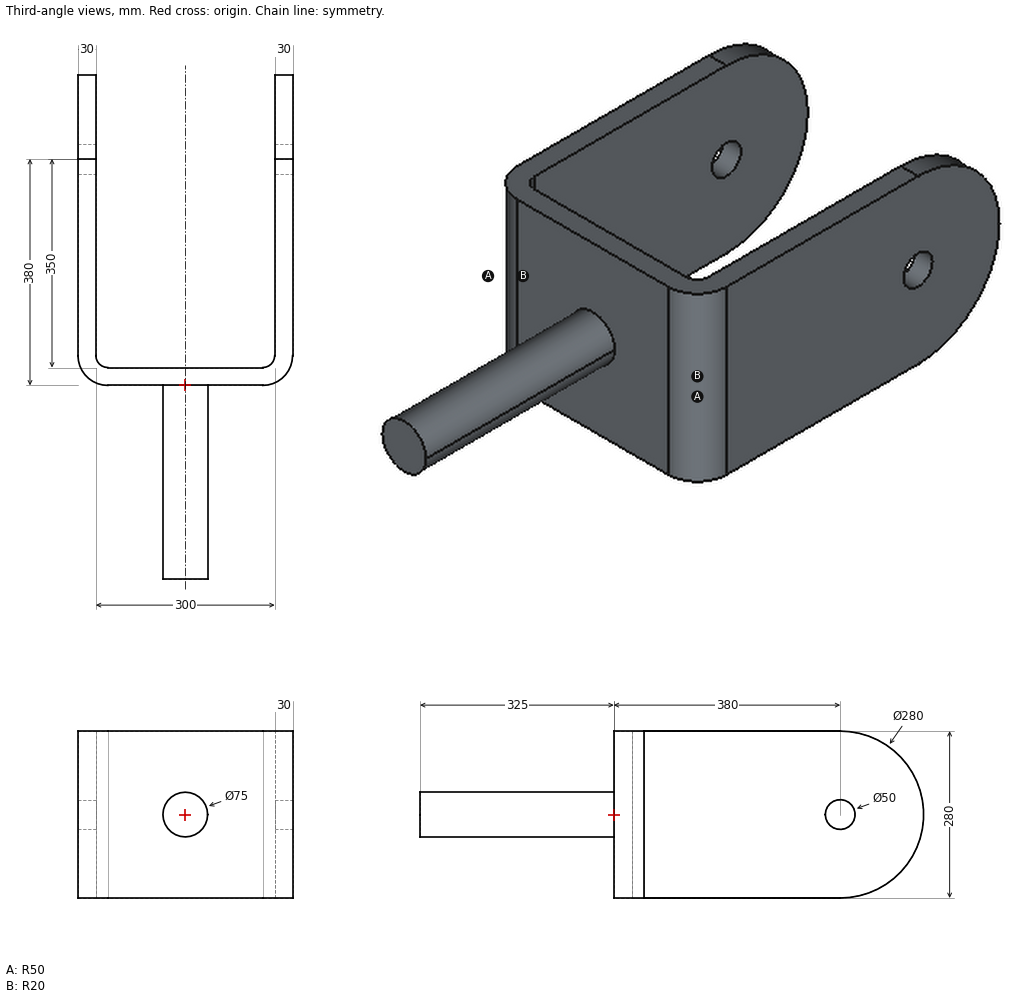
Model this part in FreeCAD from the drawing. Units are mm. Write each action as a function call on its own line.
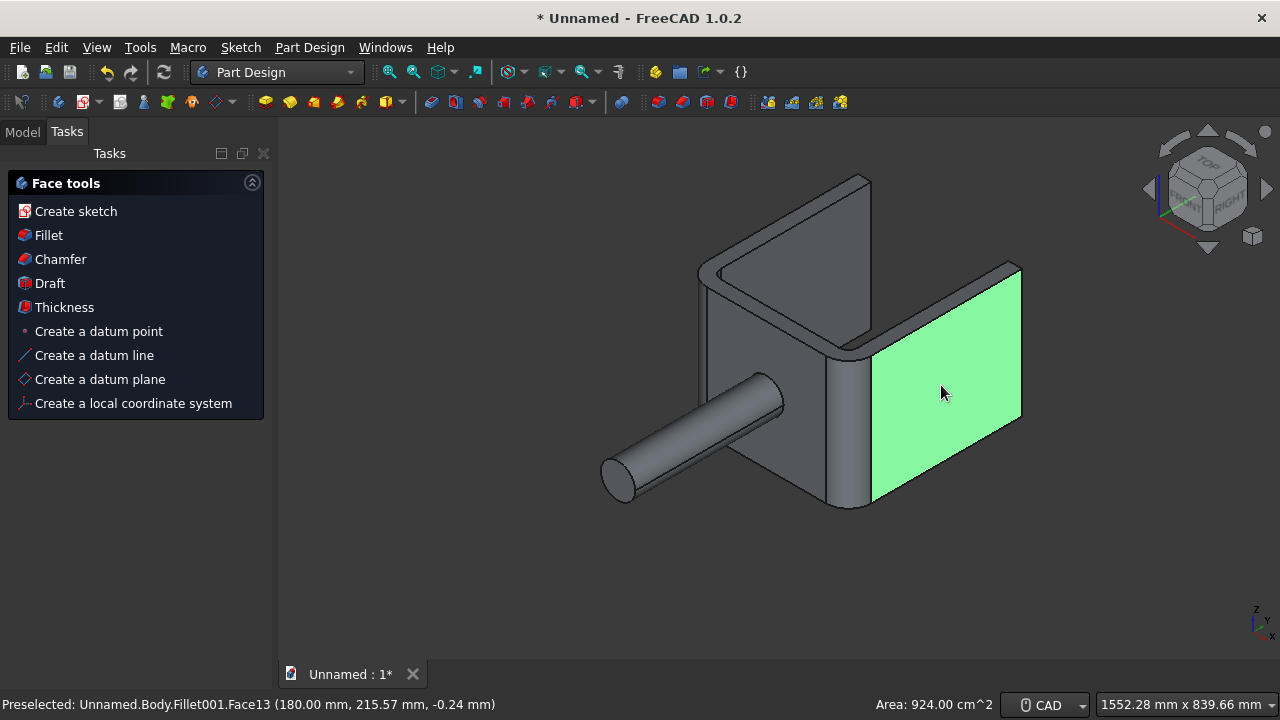
click(84, 102)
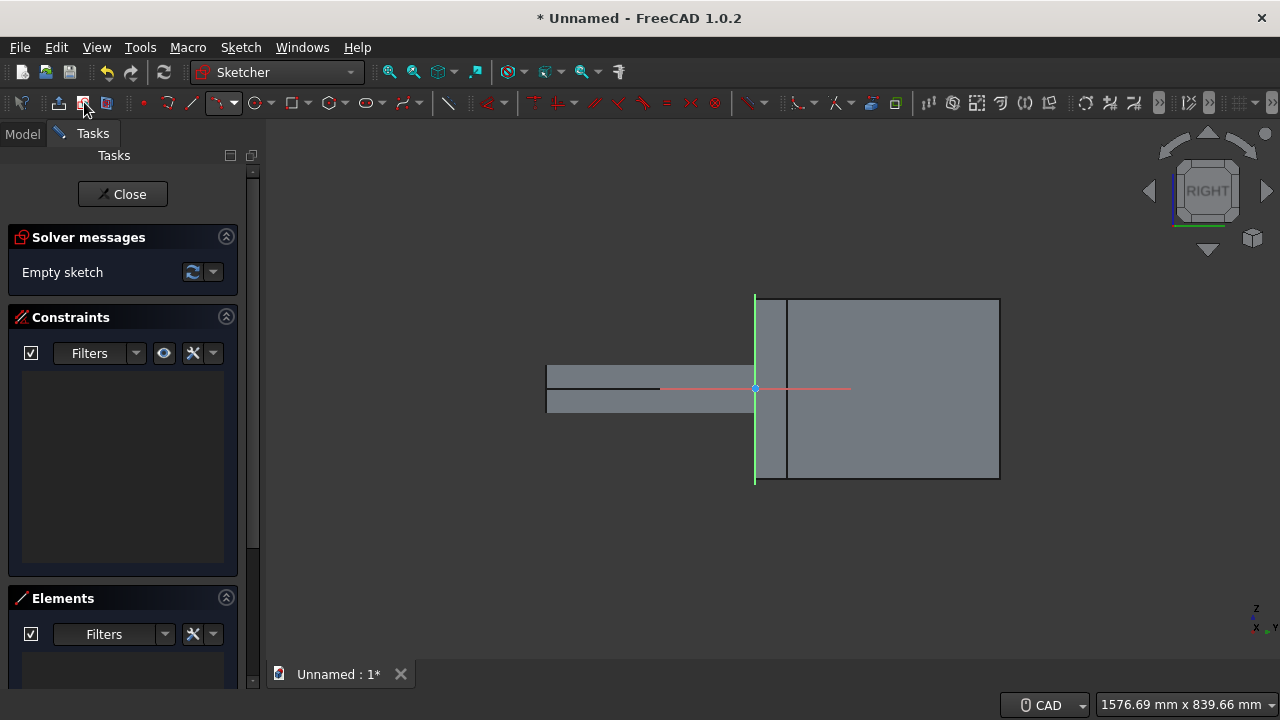
scroll(1115, 389, up, 3)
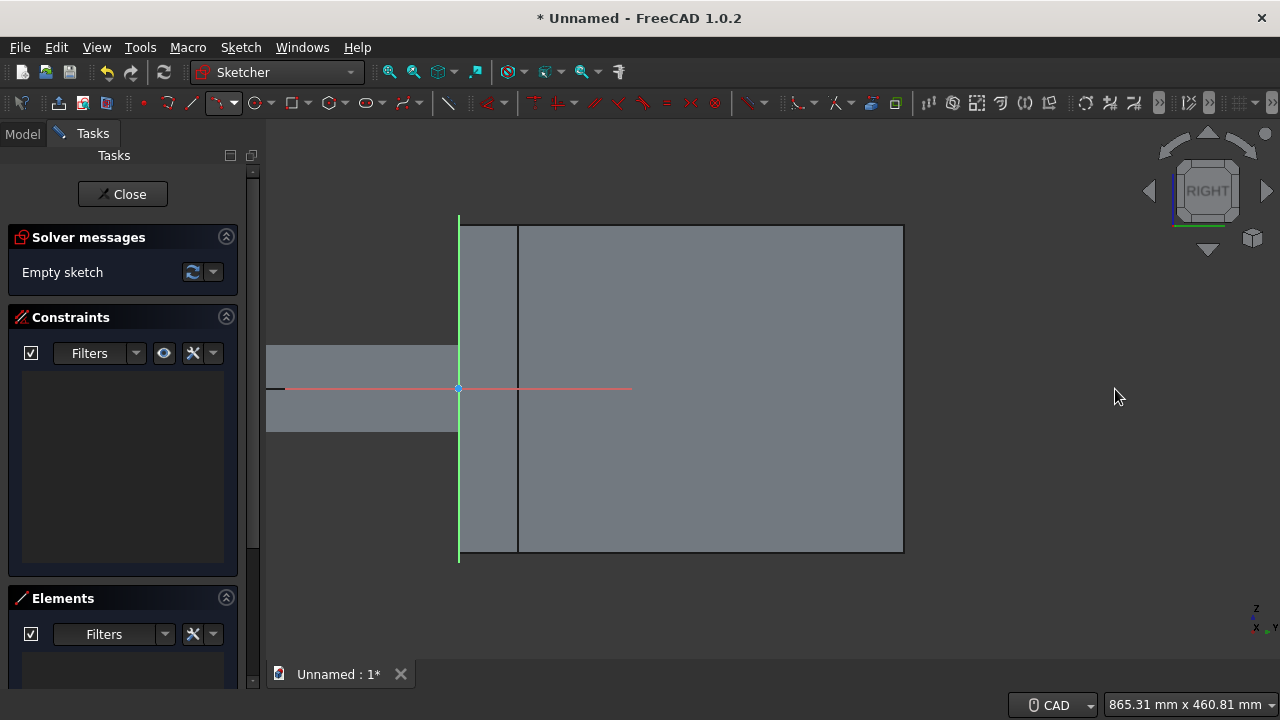
click(256, 104)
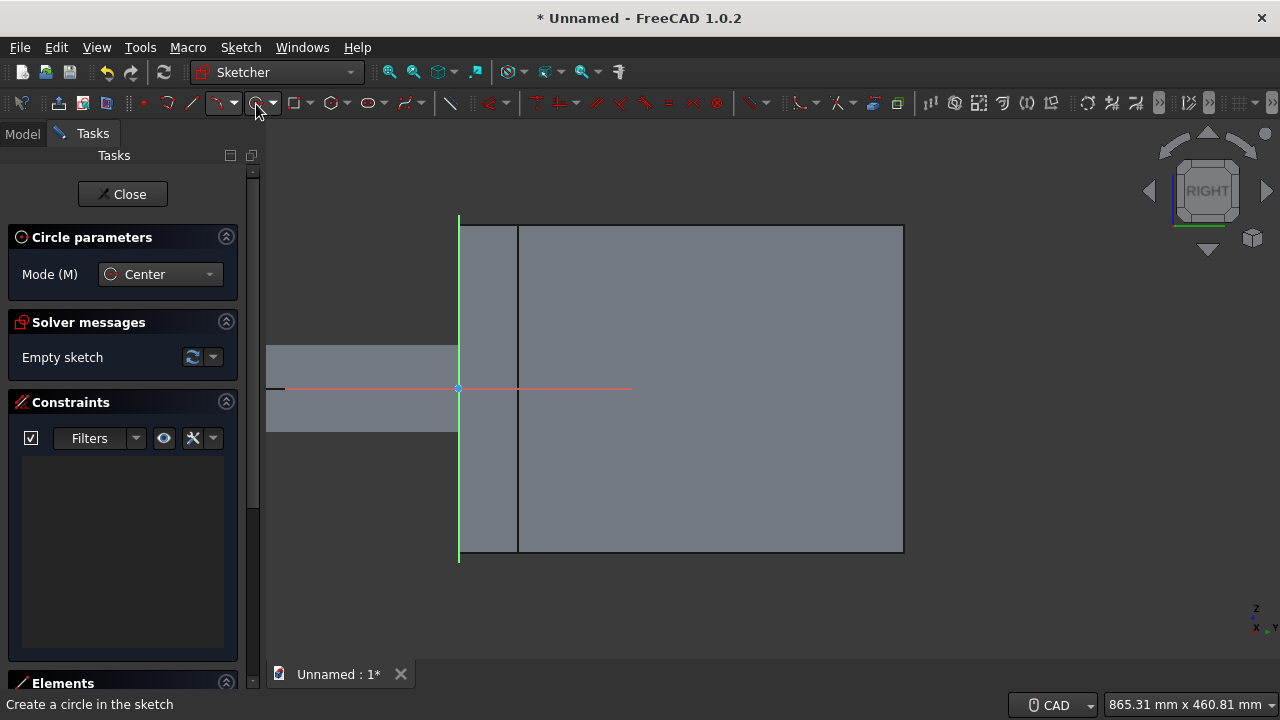
click(904, 389)
move(1020, 273)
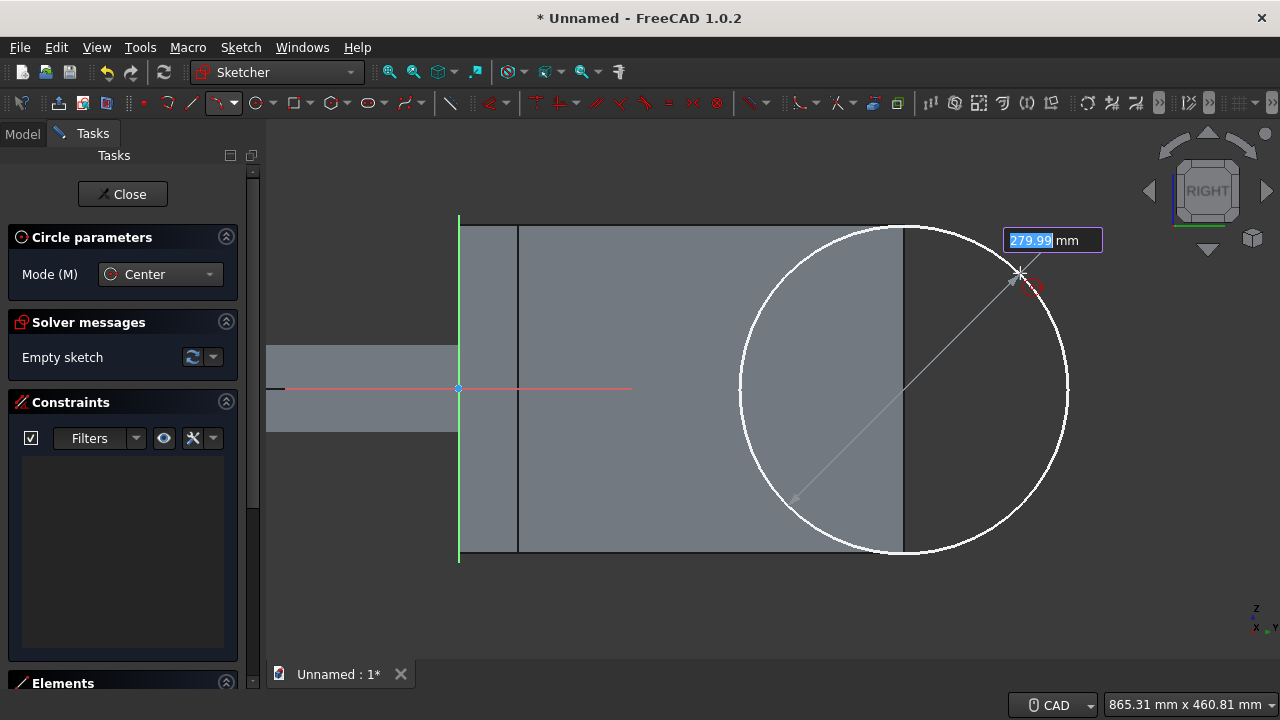
text(280)
key(Return)
key(Escape)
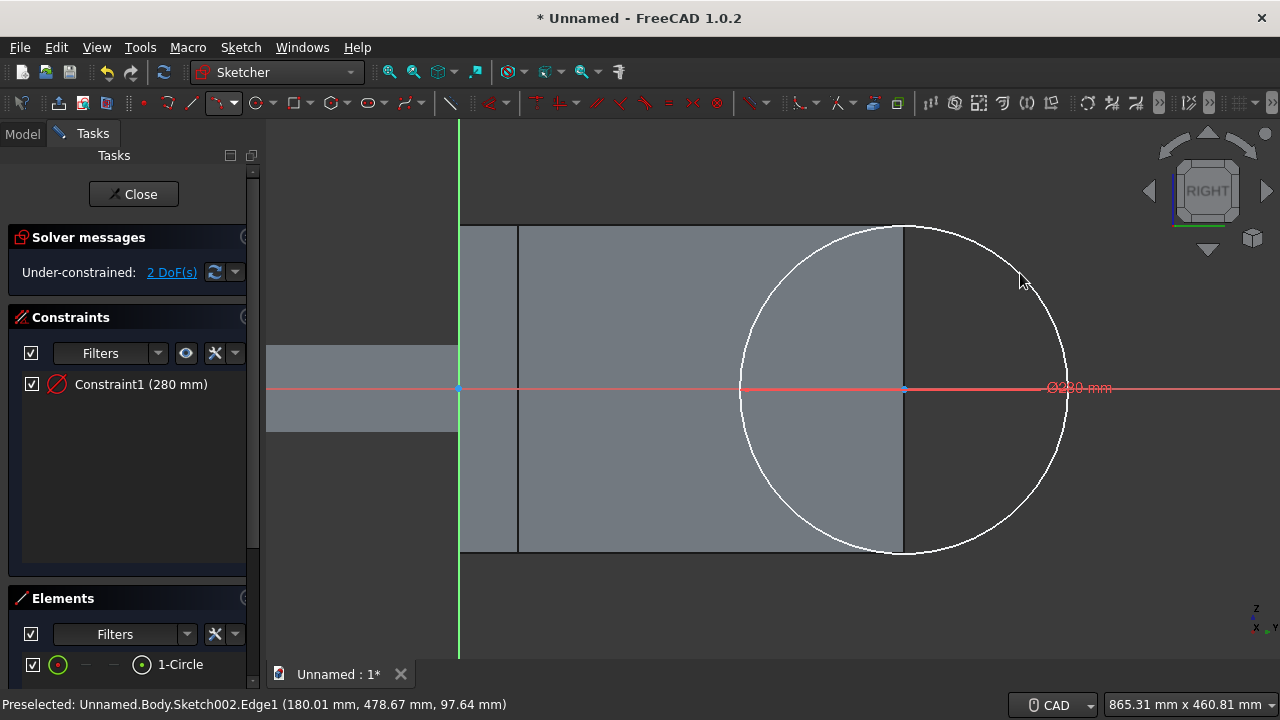
click(904, 390)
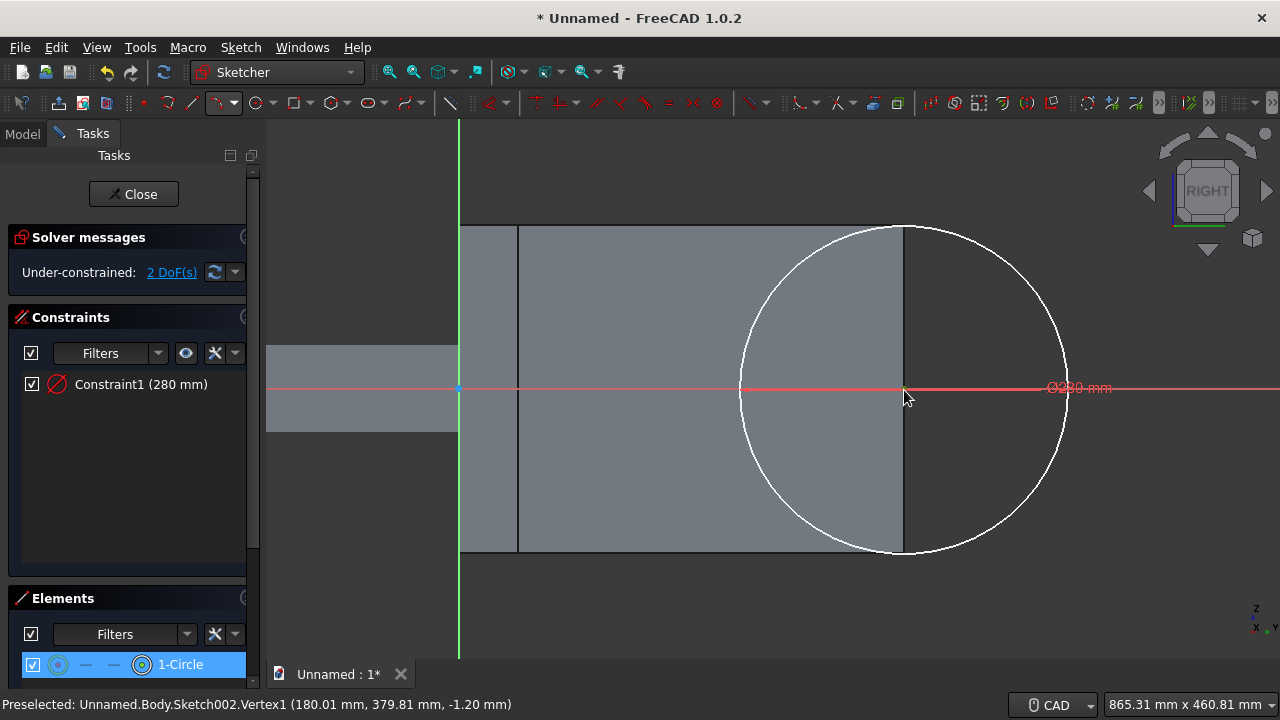
click(353, 389)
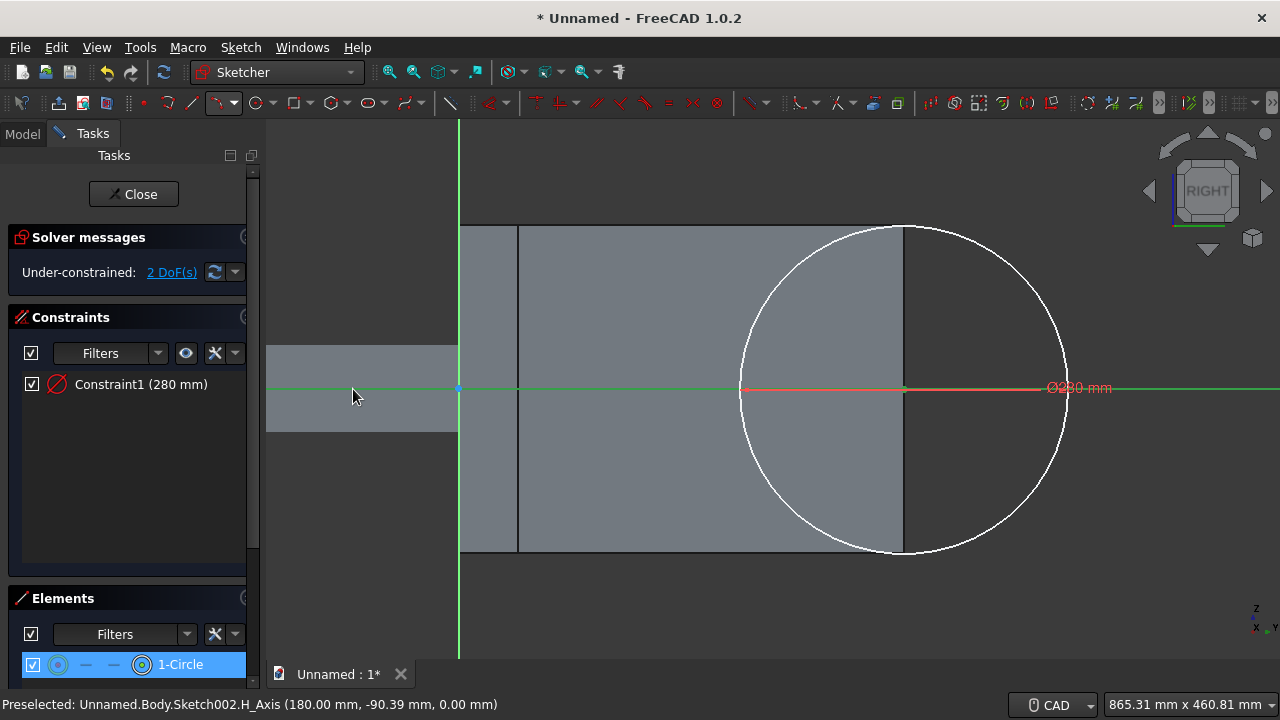
click(536, 104)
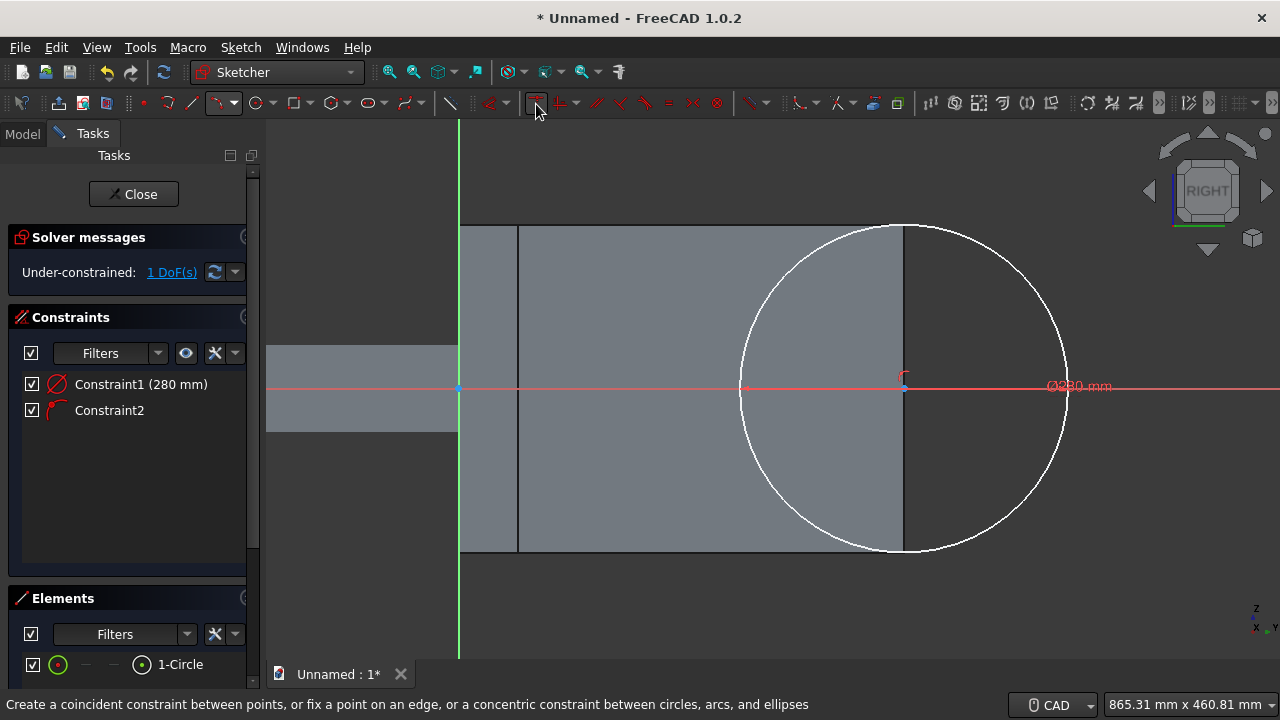
click(490, 104)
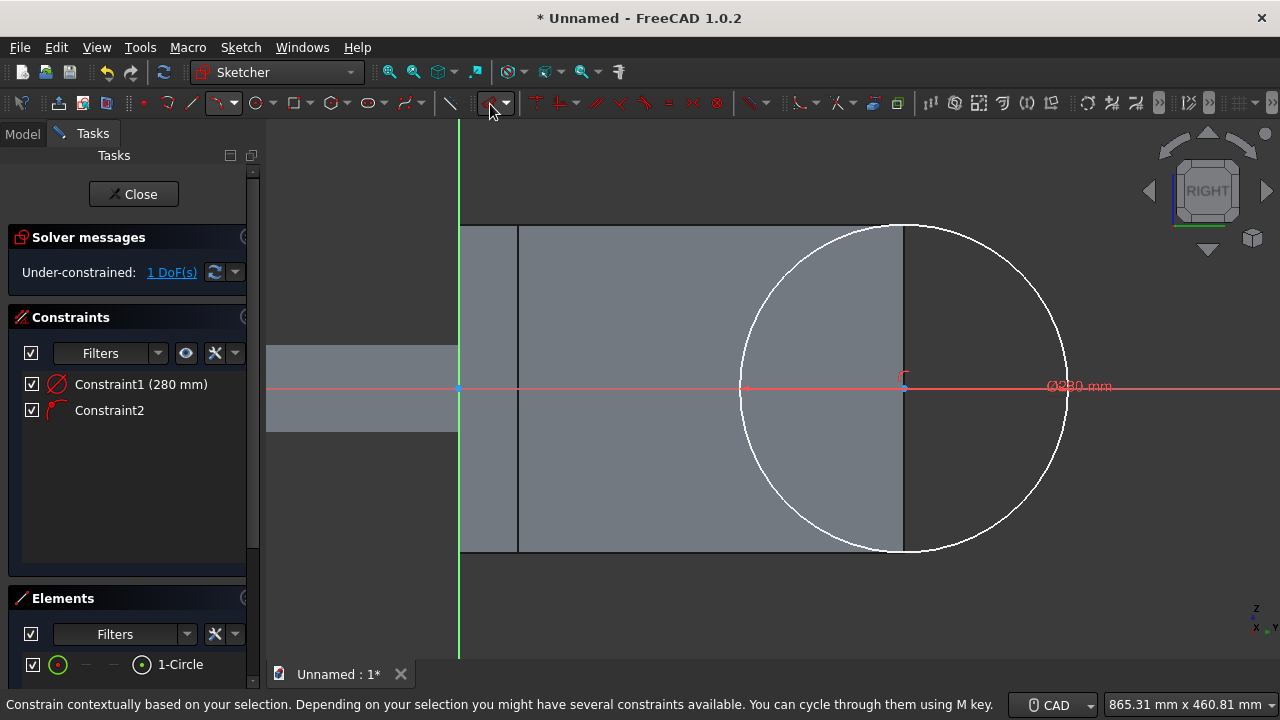
click(904, 389)
click(681, 423)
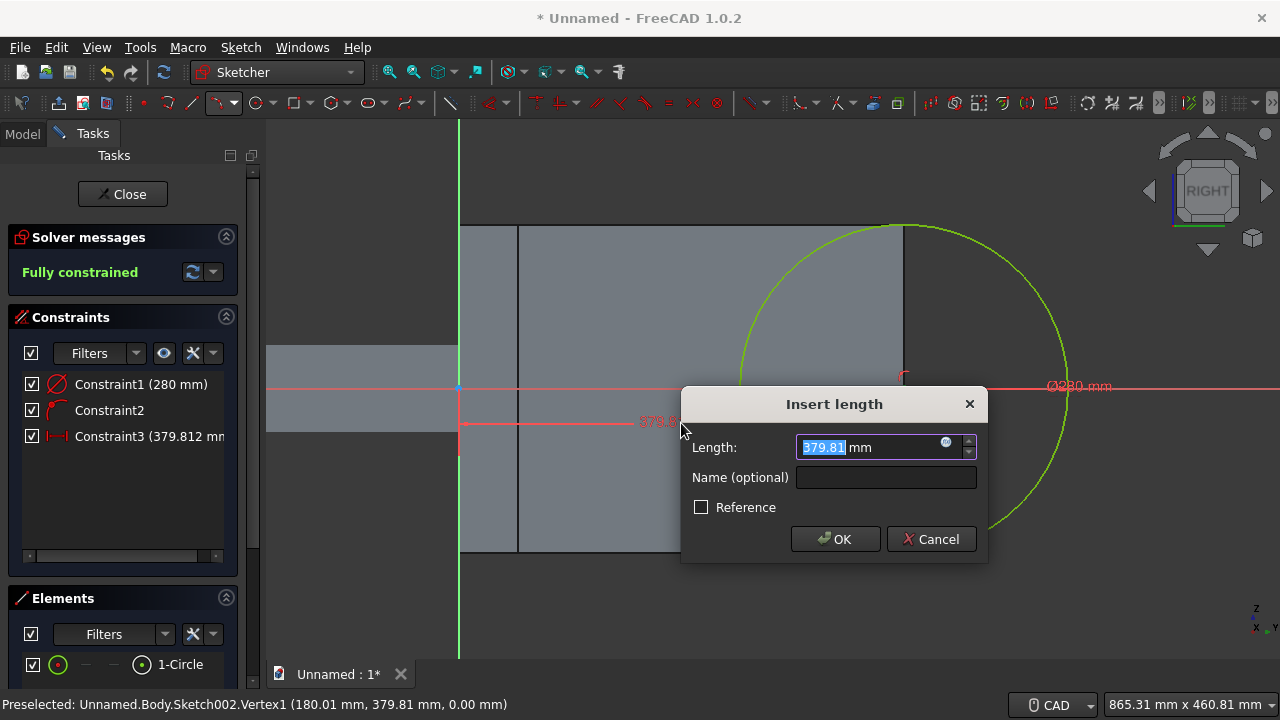
text(380)
key(Return)
key(Escape)